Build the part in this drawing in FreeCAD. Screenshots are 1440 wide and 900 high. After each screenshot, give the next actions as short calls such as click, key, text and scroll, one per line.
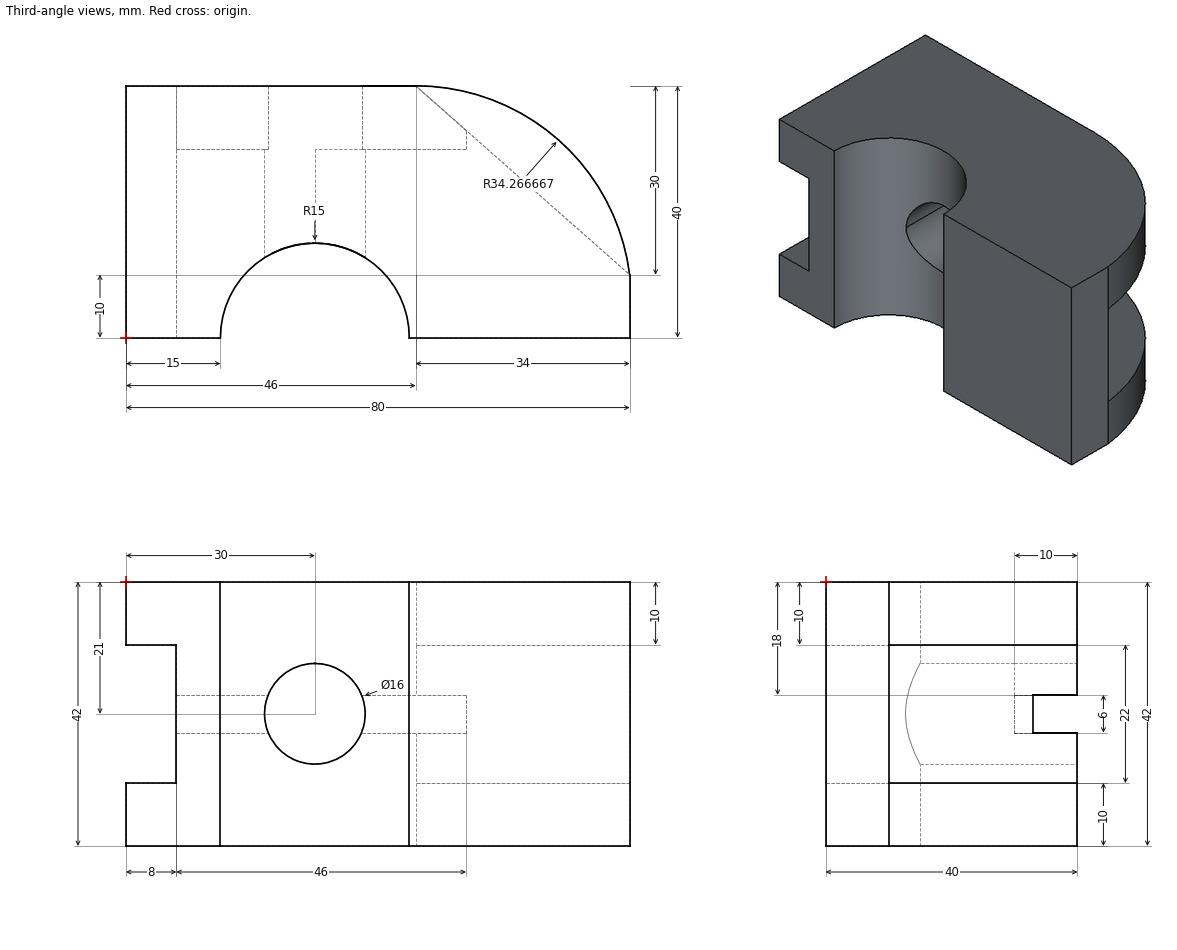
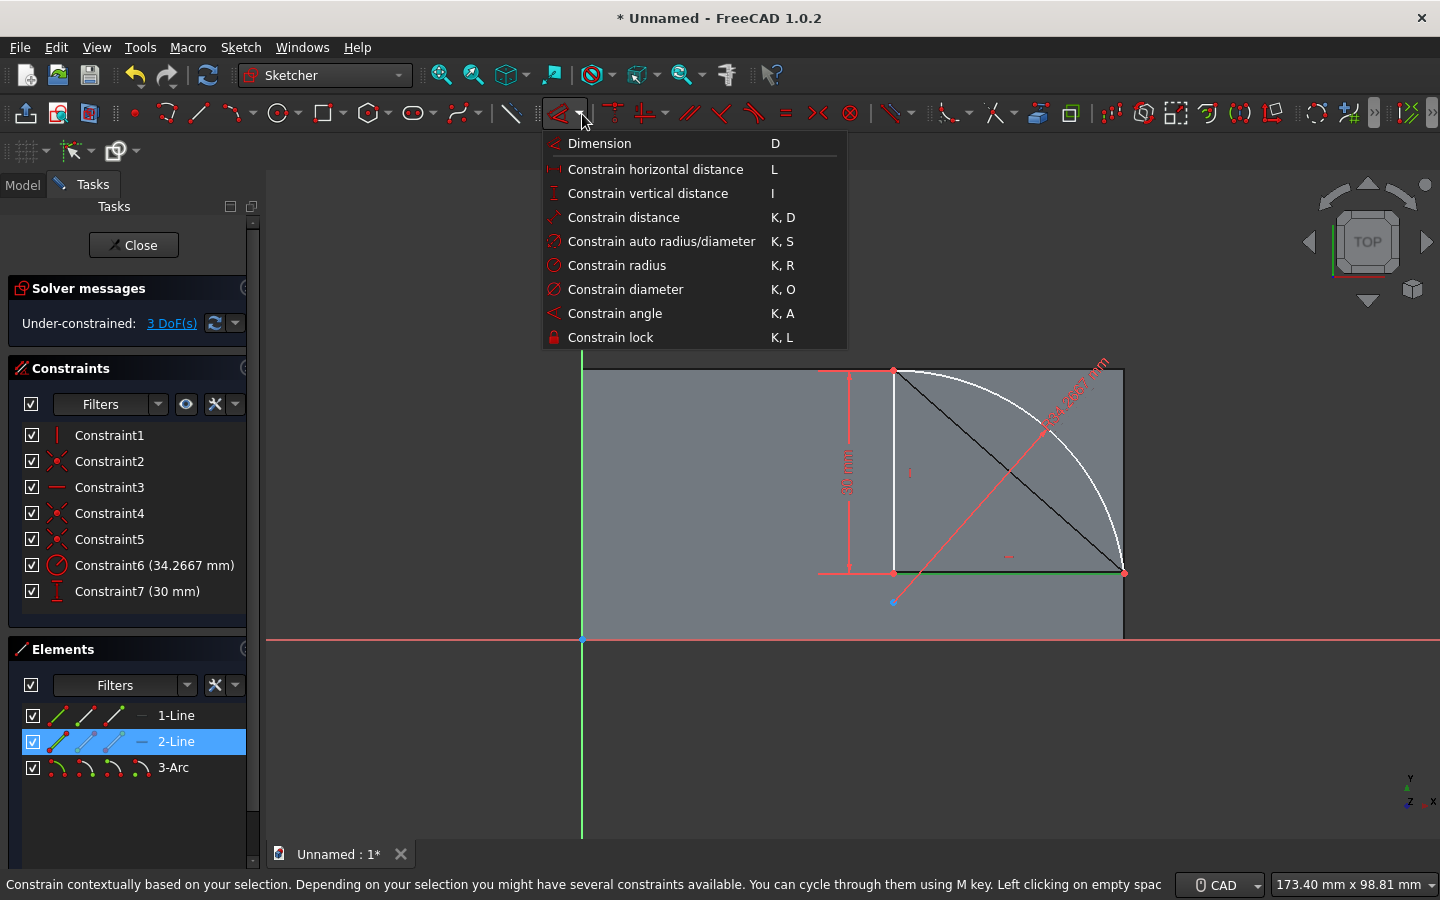
click(695, 169)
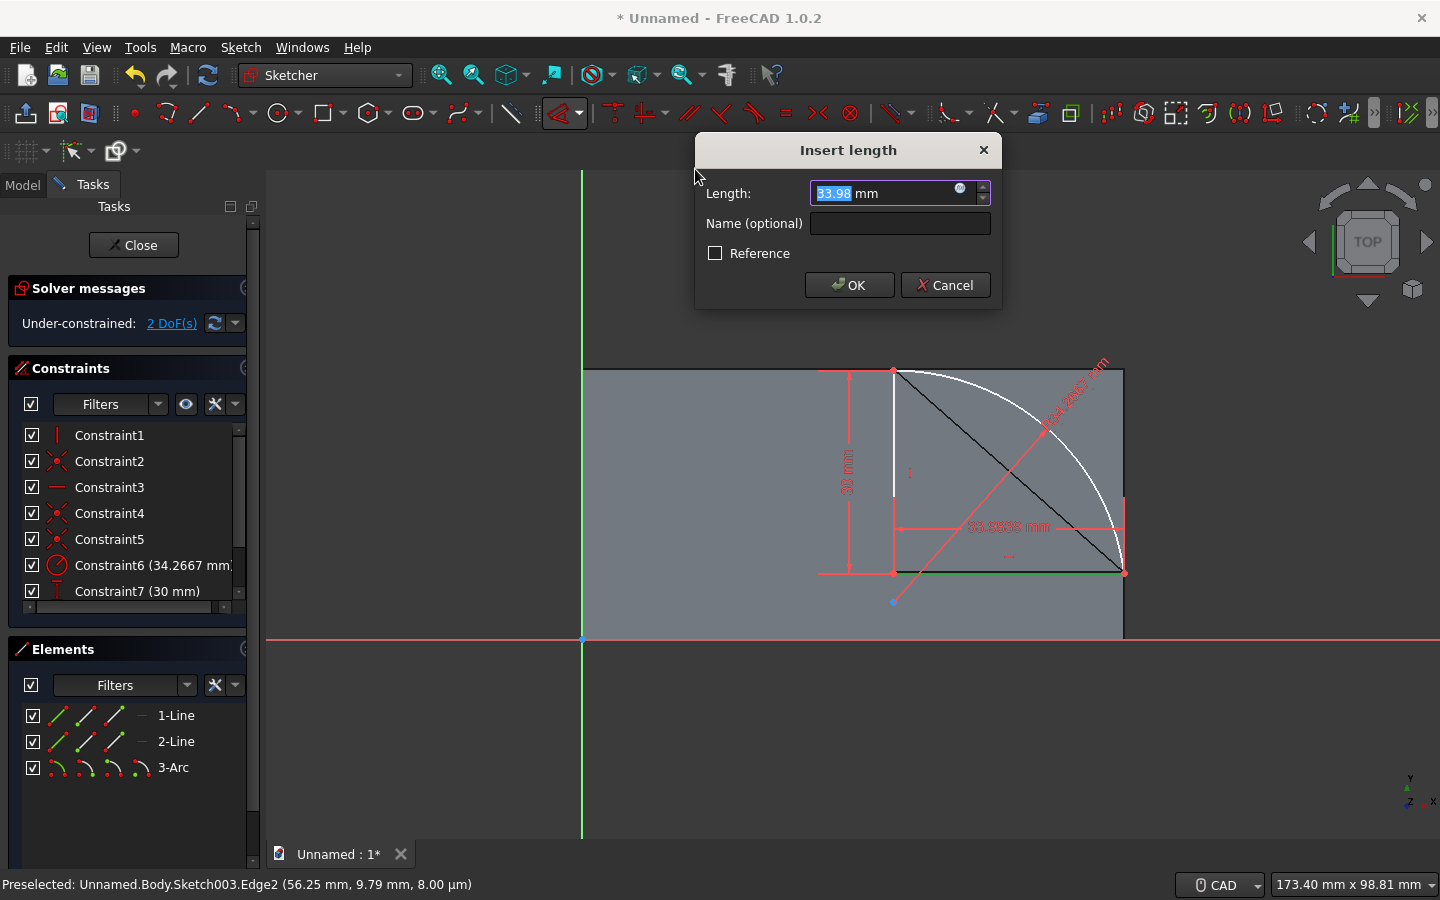
text(34)
key(Return)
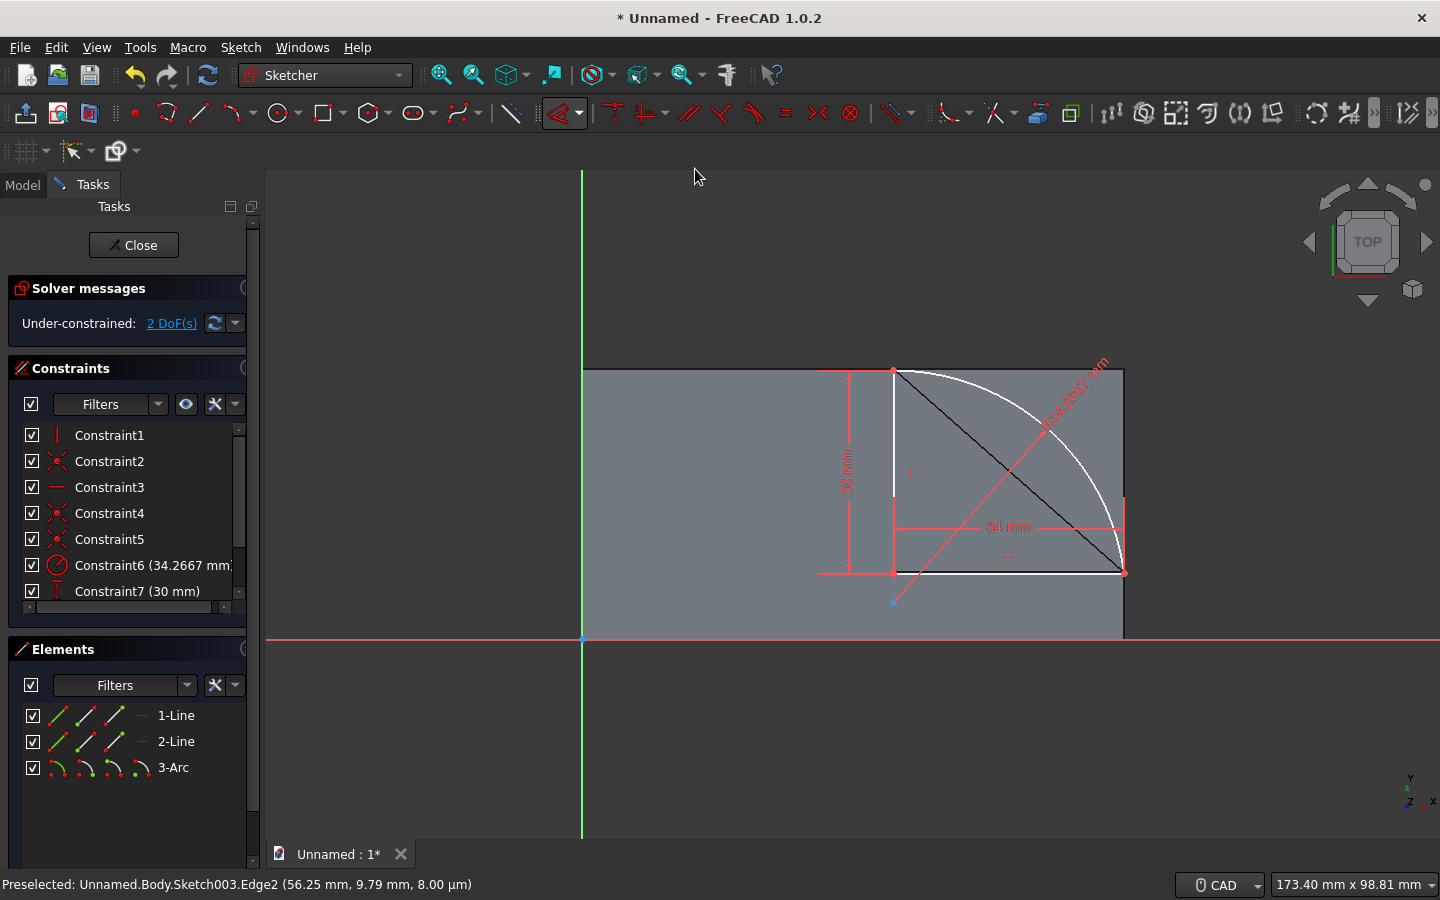
click(894, 371)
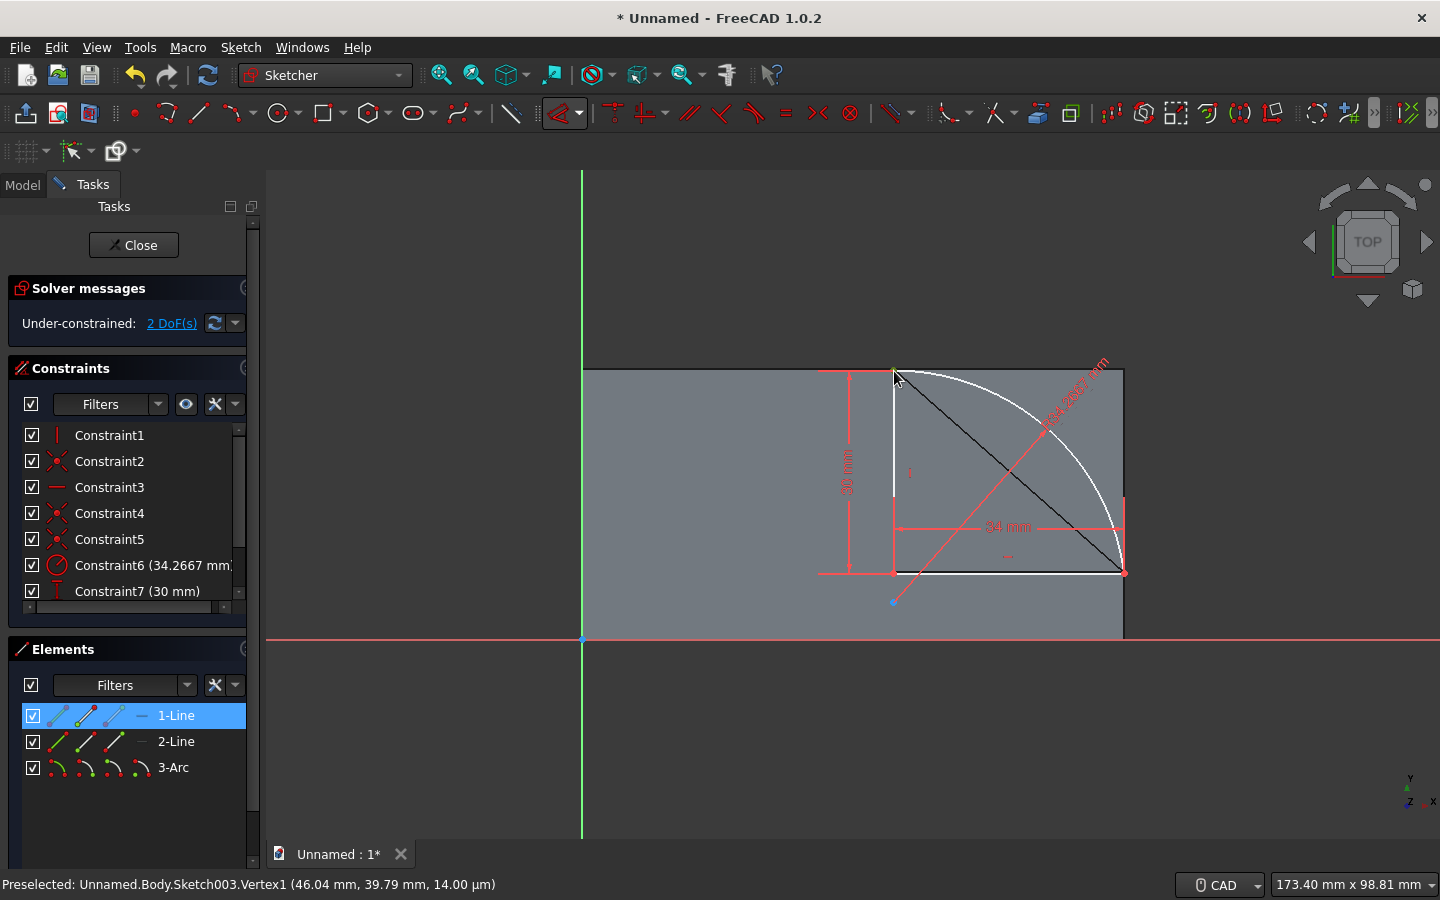
click(582, 114)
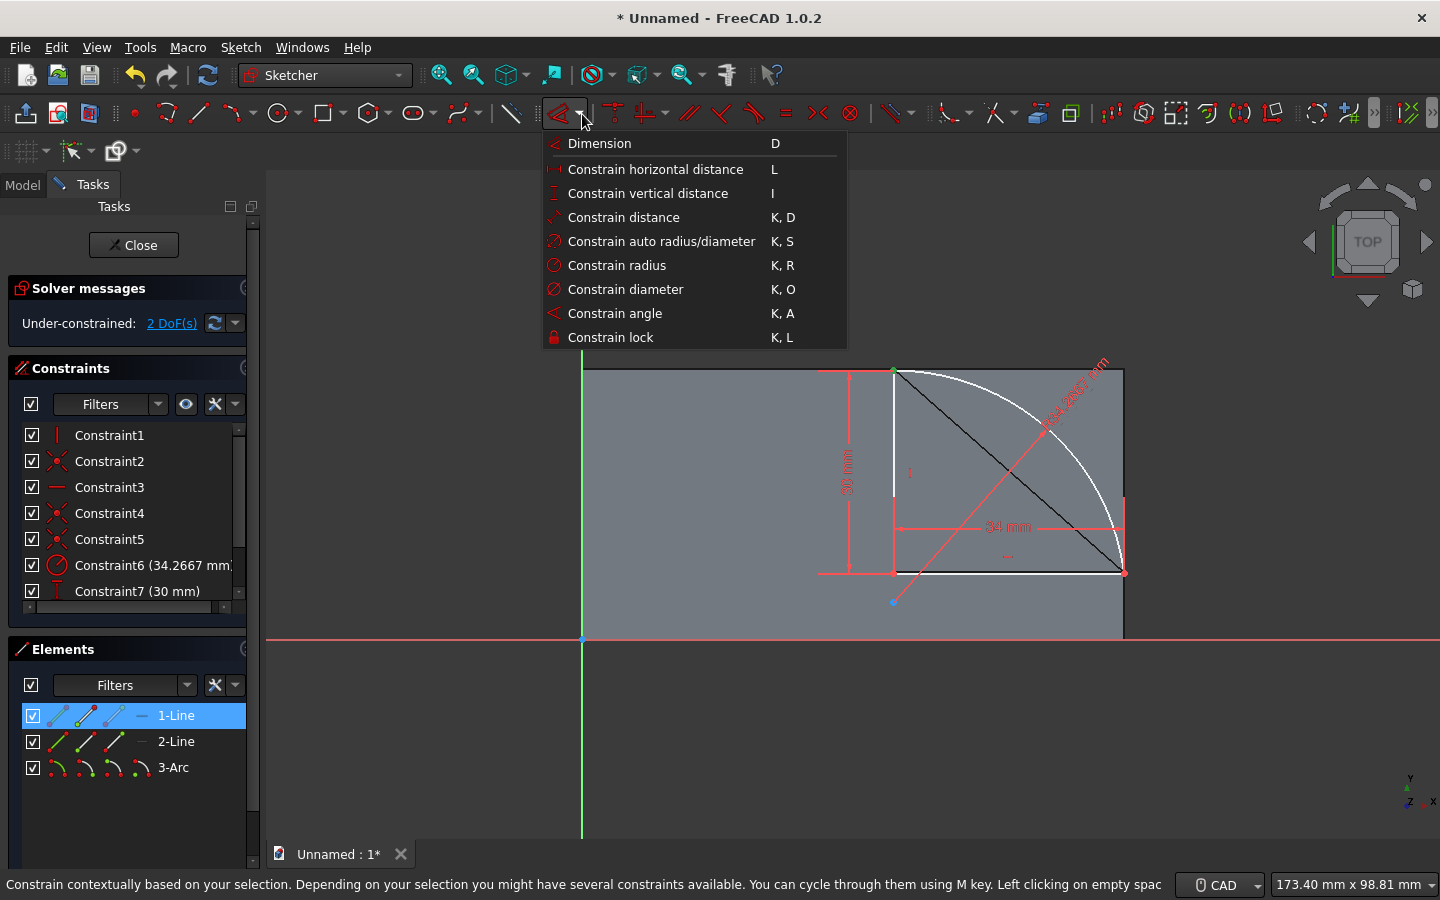
click(695, 169)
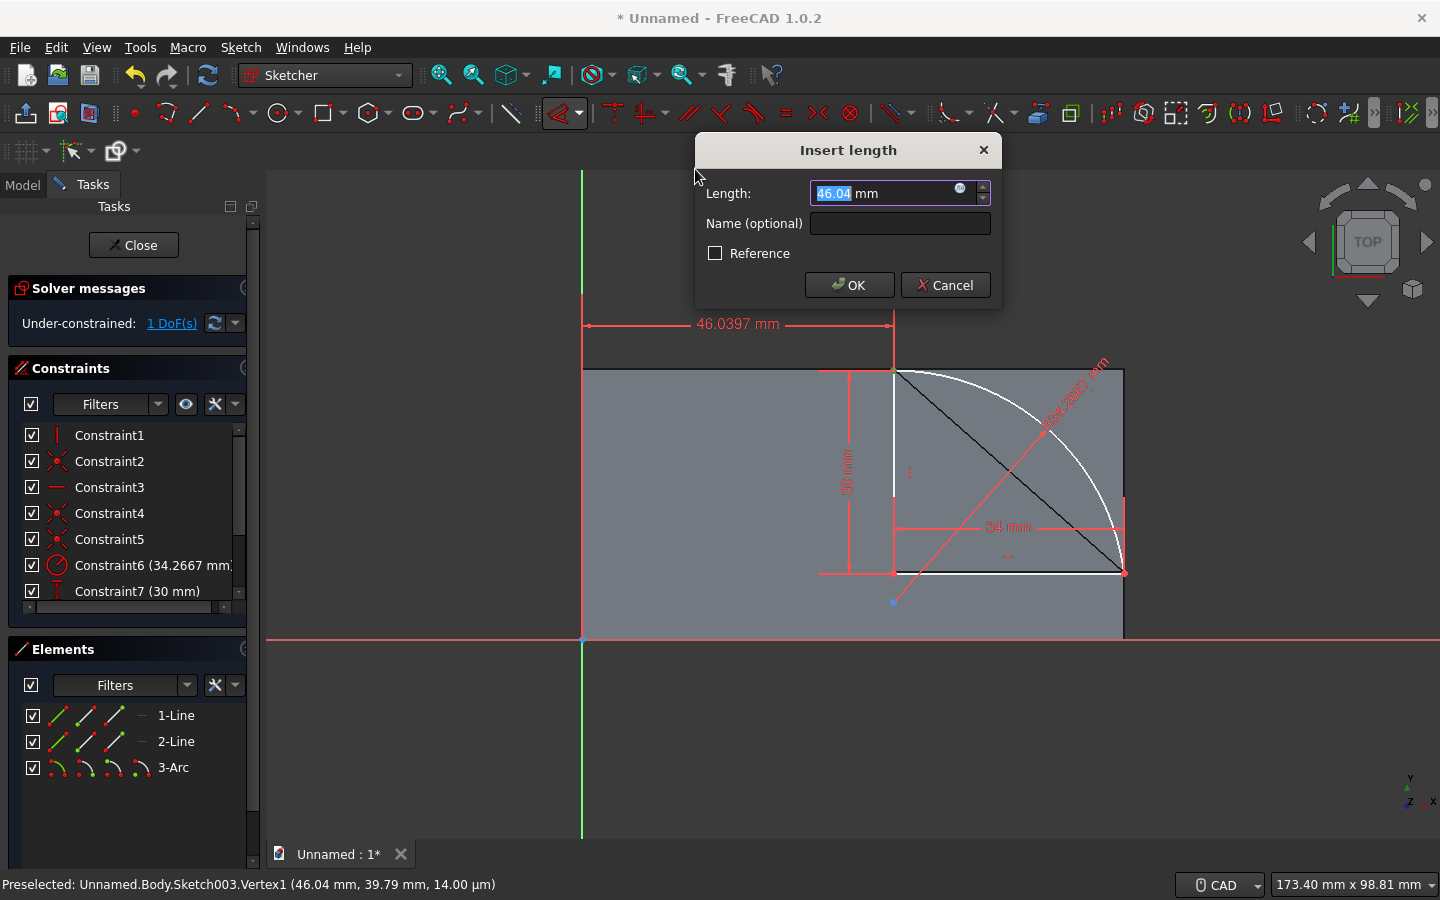
text(46)
key(Return)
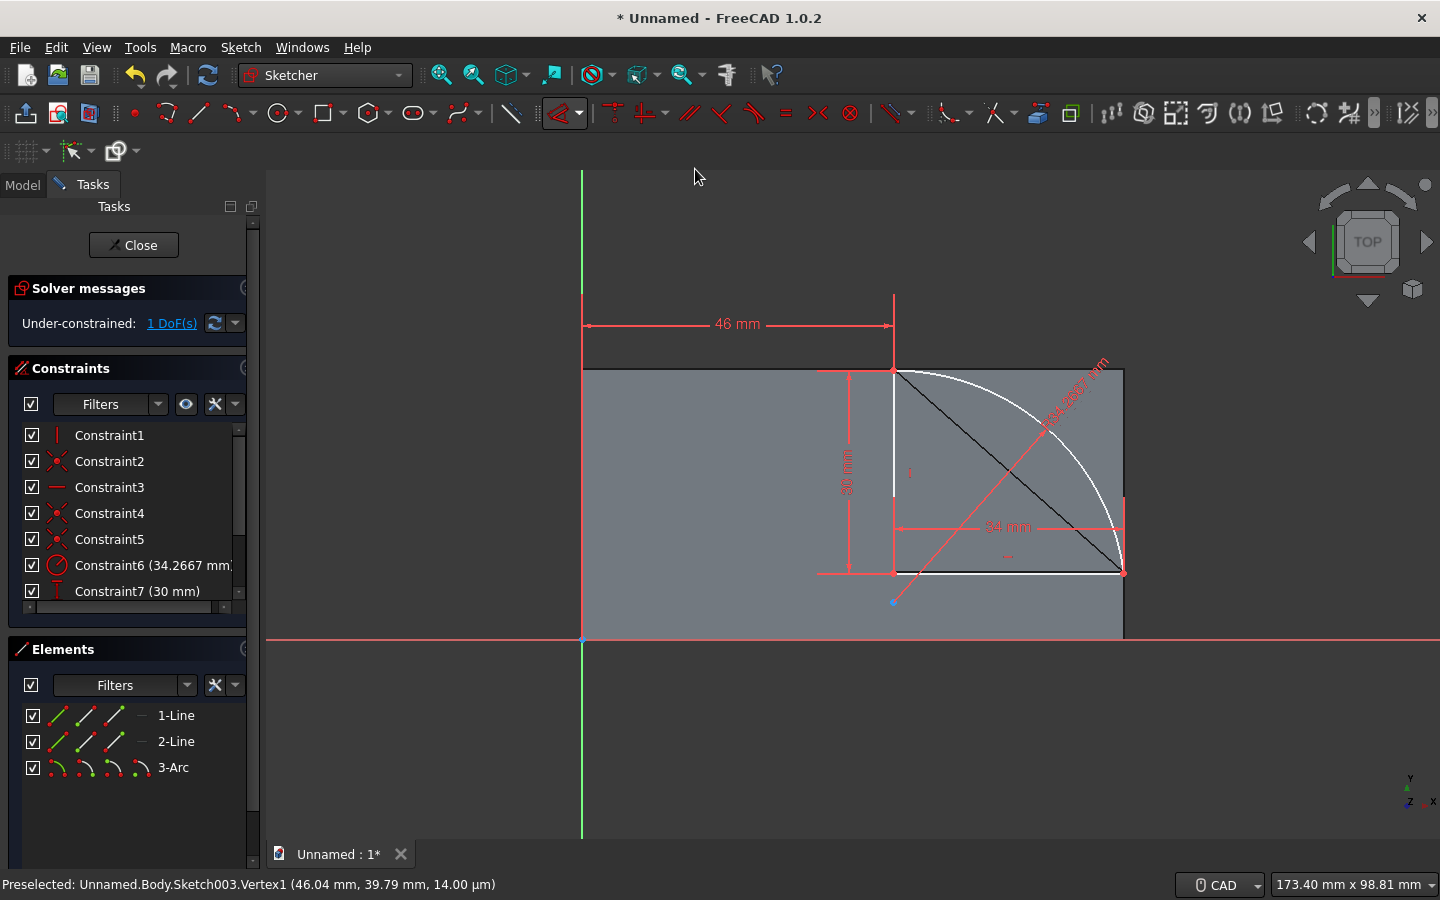
click(894, 371)